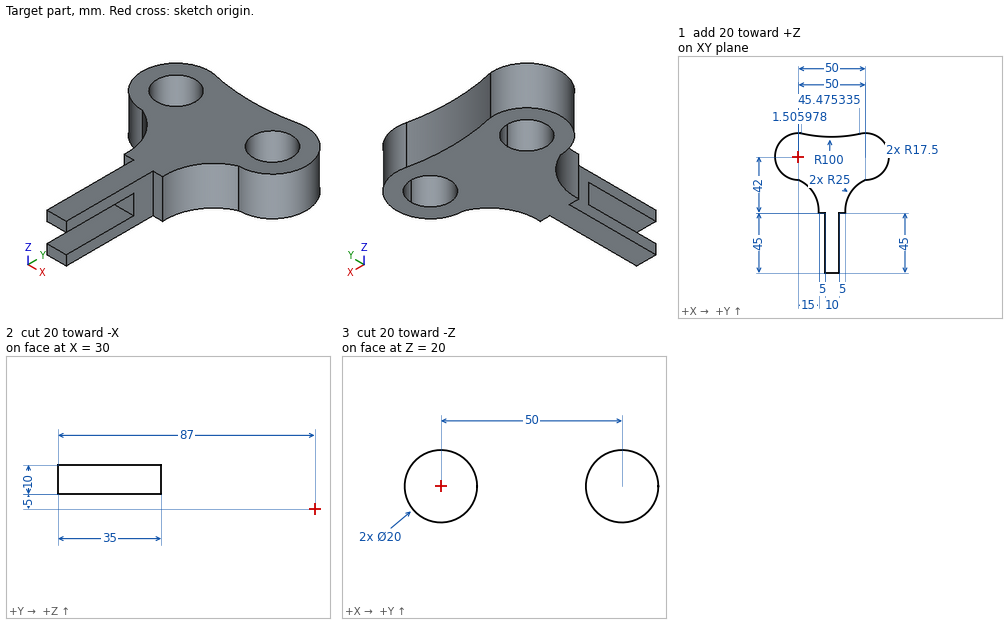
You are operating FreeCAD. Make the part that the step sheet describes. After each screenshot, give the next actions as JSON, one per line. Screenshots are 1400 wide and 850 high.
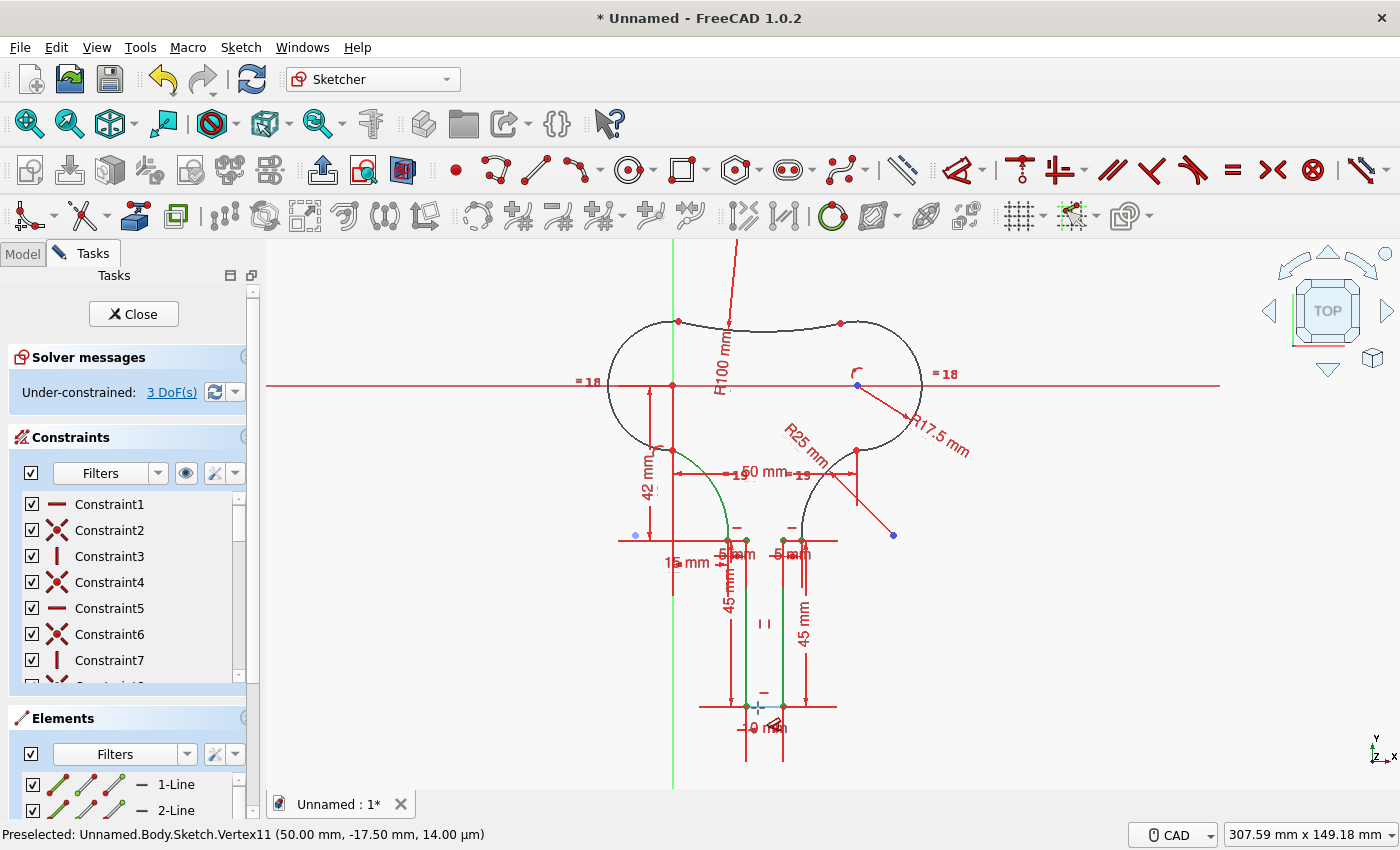
{"action": "left_click", "coordinate": [857, 386]}
{"action": "left_click", "coordinate": [807, 352]}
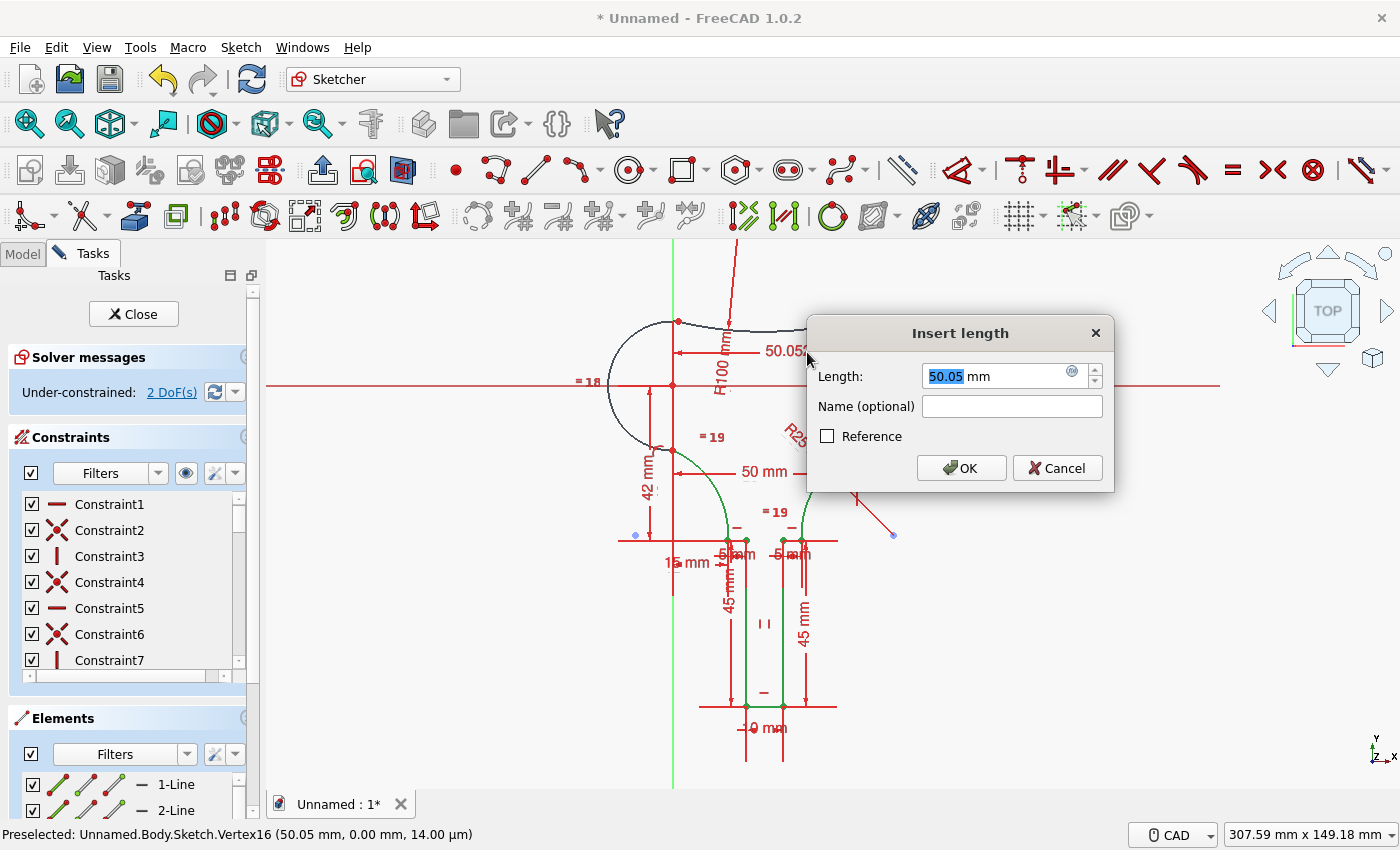
{"action": "type", "text": "50"}
{"action": "key", "text": "Return"}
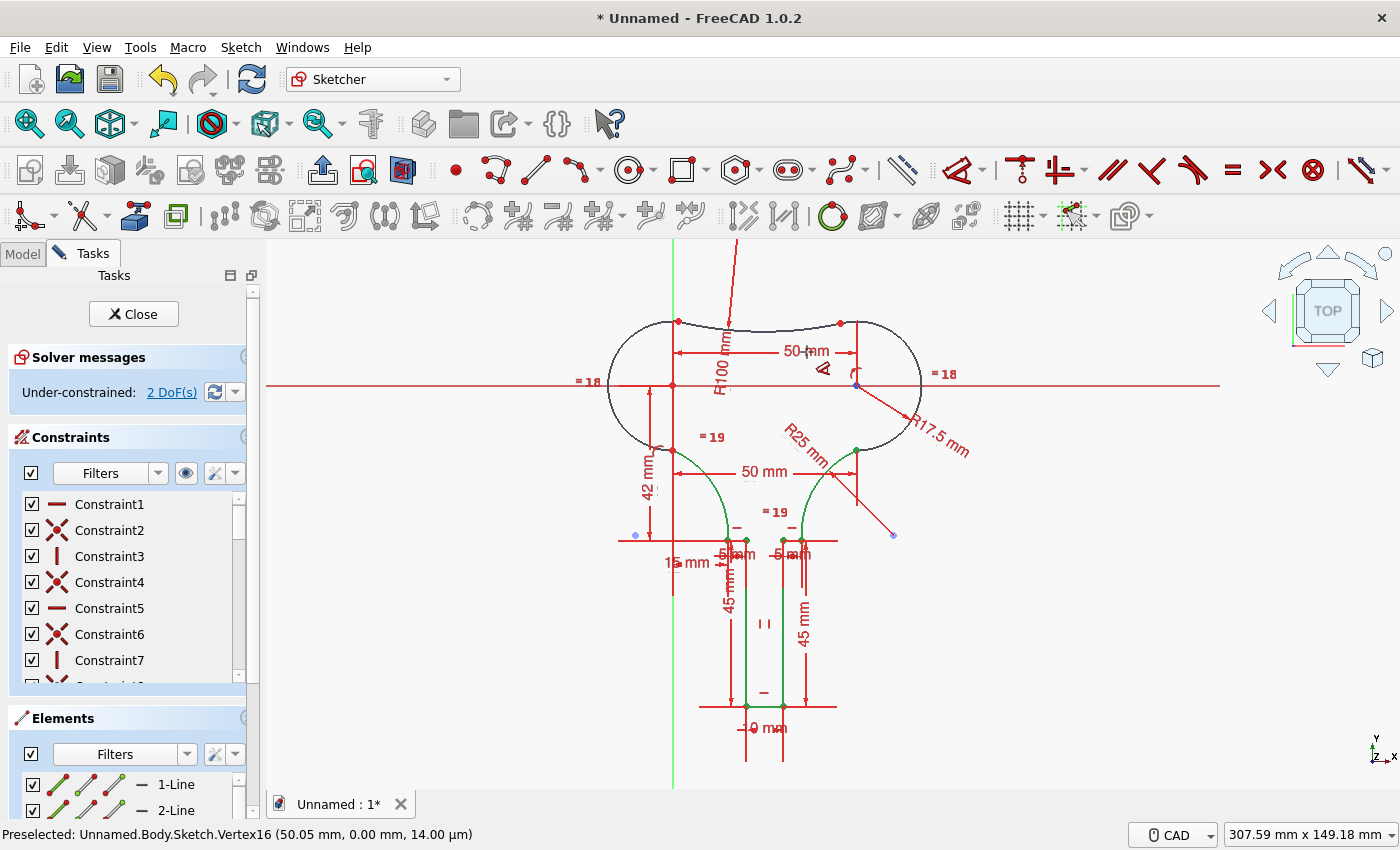
{"action": "scroll", "coordinate": [678, 322], "scroll_direction": "up", "scroll_amount": 10}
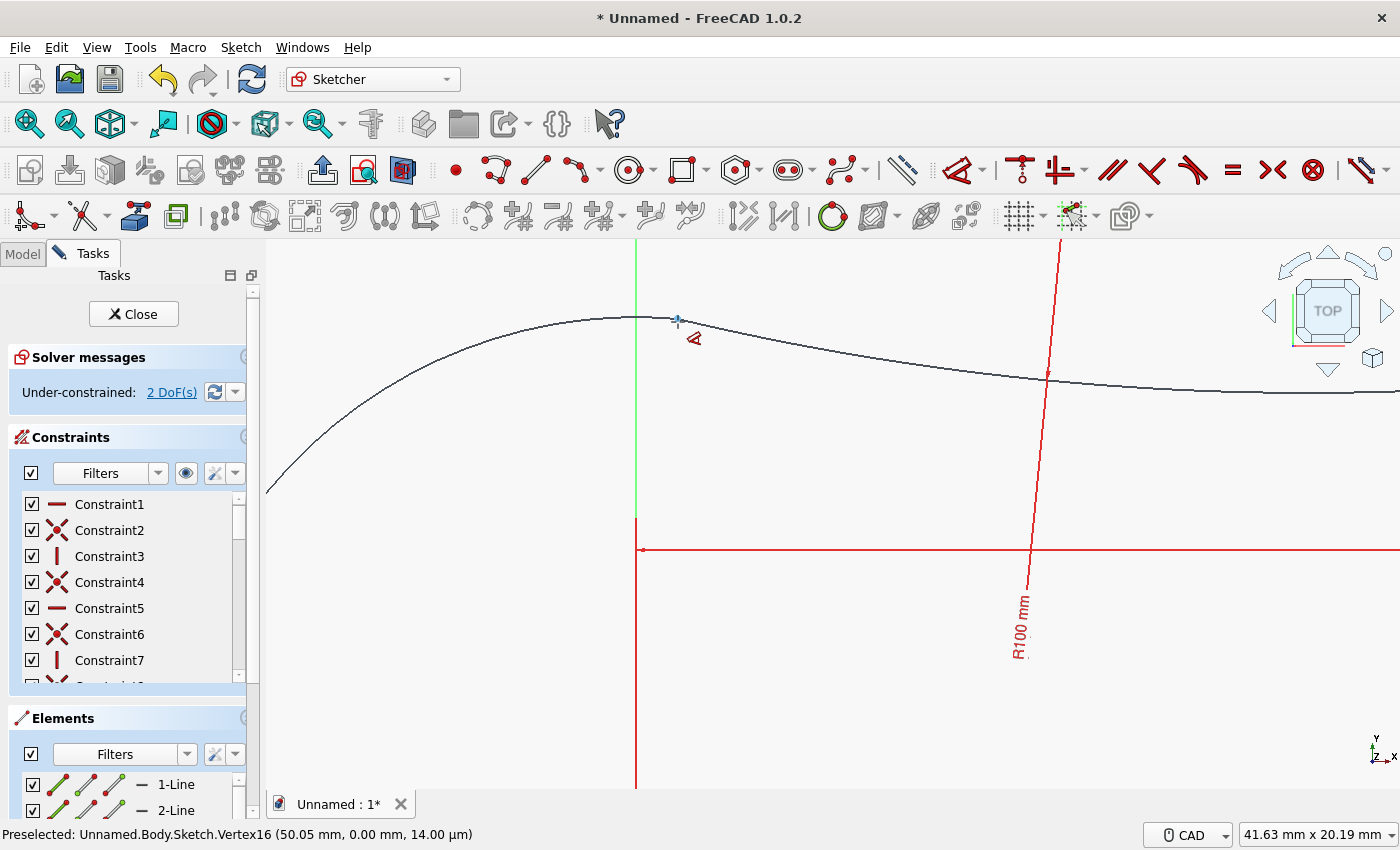
{"action": "left_click", "coordinate": [677, 319]}
{"action": "left_click", "coordinate": [657, 285]}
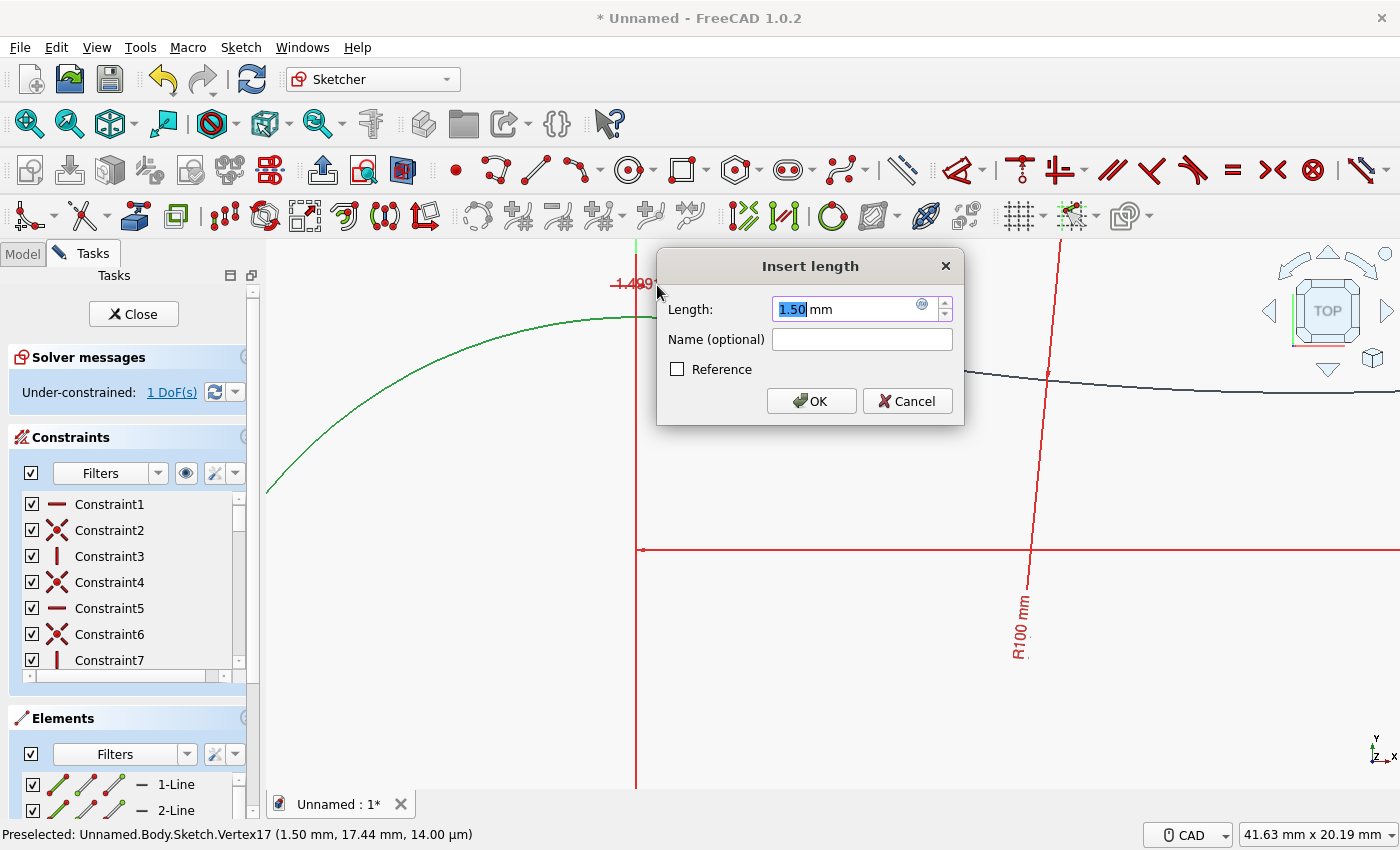
{"action": "type", "text": "1.505978"}
{"action": "key", "text": "Return"}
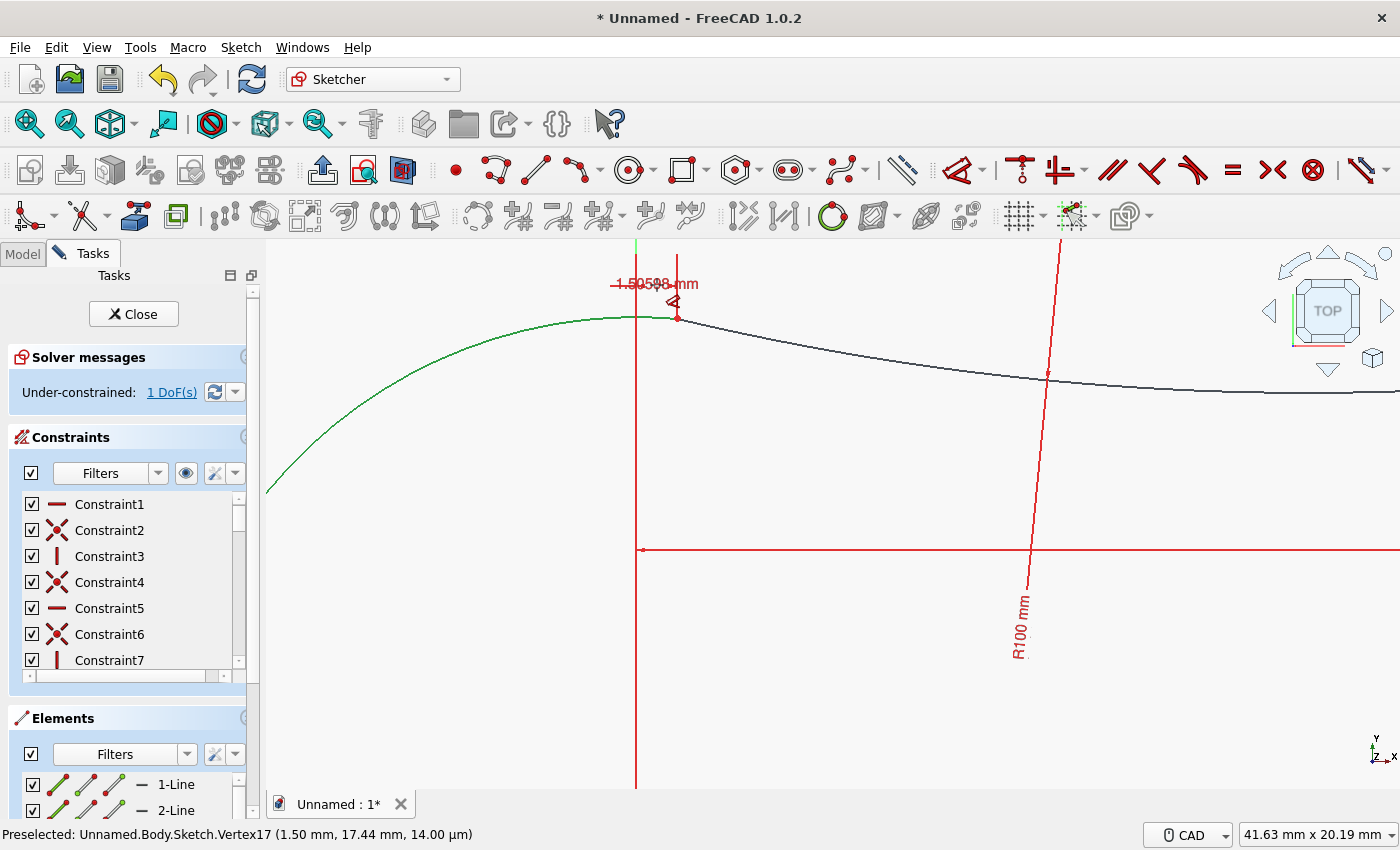
{"action": "scroll", "coordinate": [678, 322], "scroll_direction": "down", "scroll_amount": 10}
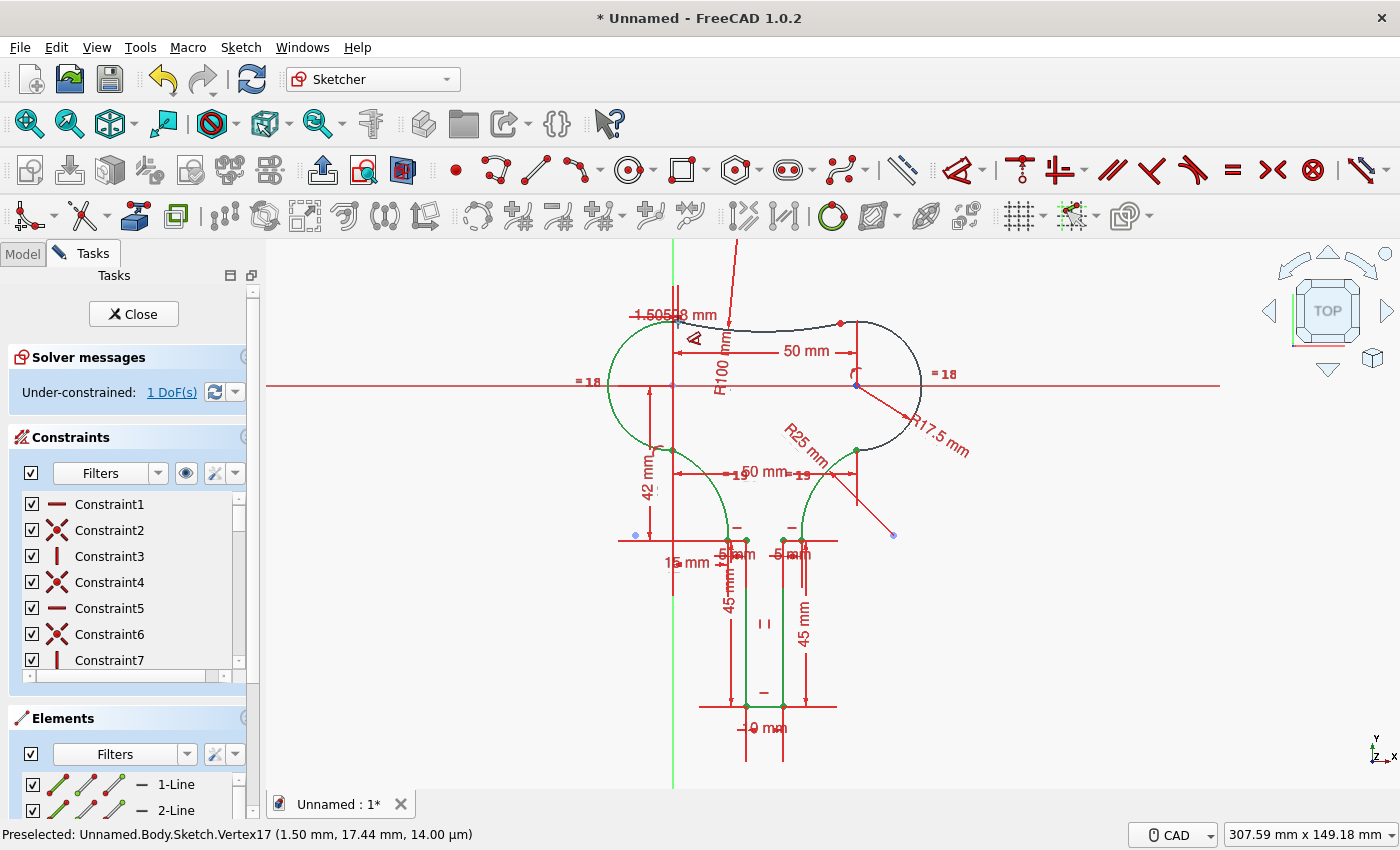
{"action": "left_click", "coordinate": [841, 324]}
{"action": "left_click", "coordinate": [757, 290]}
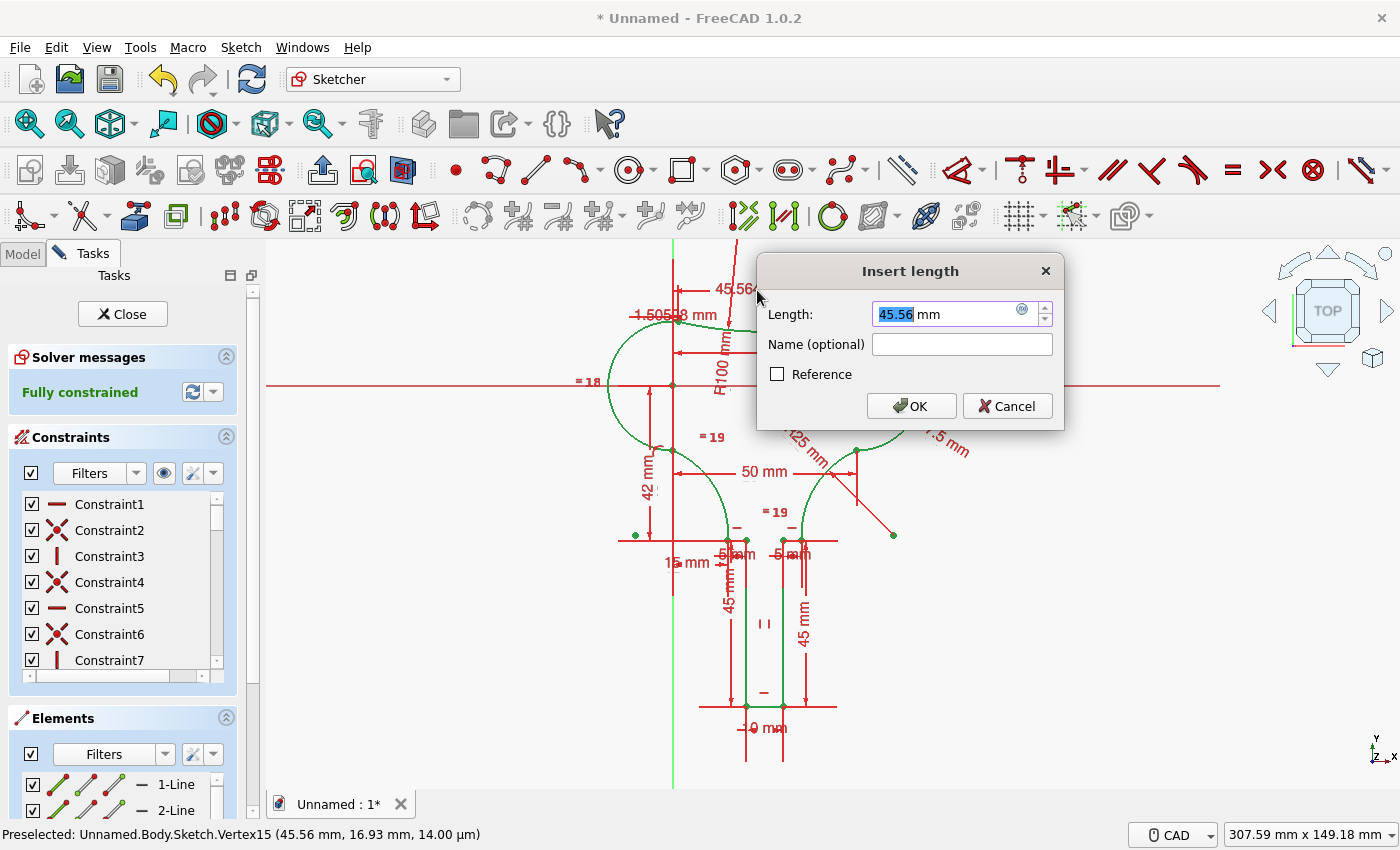
{"action": "type", "text": "45.475335"}
{"action": "key", "text": "Return"}
{"action": "key", "text": "Escape"}